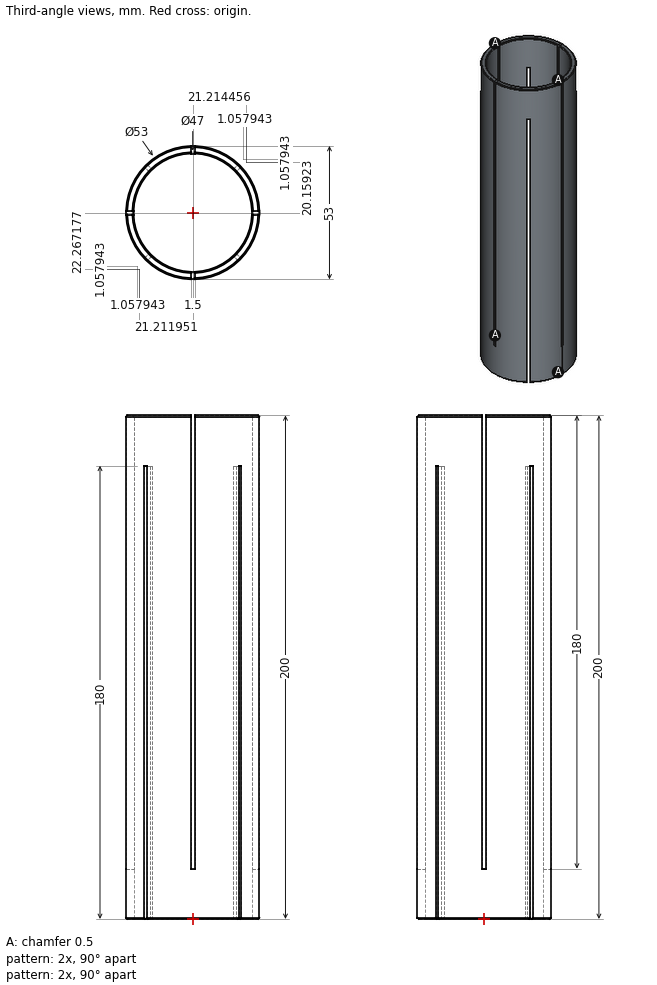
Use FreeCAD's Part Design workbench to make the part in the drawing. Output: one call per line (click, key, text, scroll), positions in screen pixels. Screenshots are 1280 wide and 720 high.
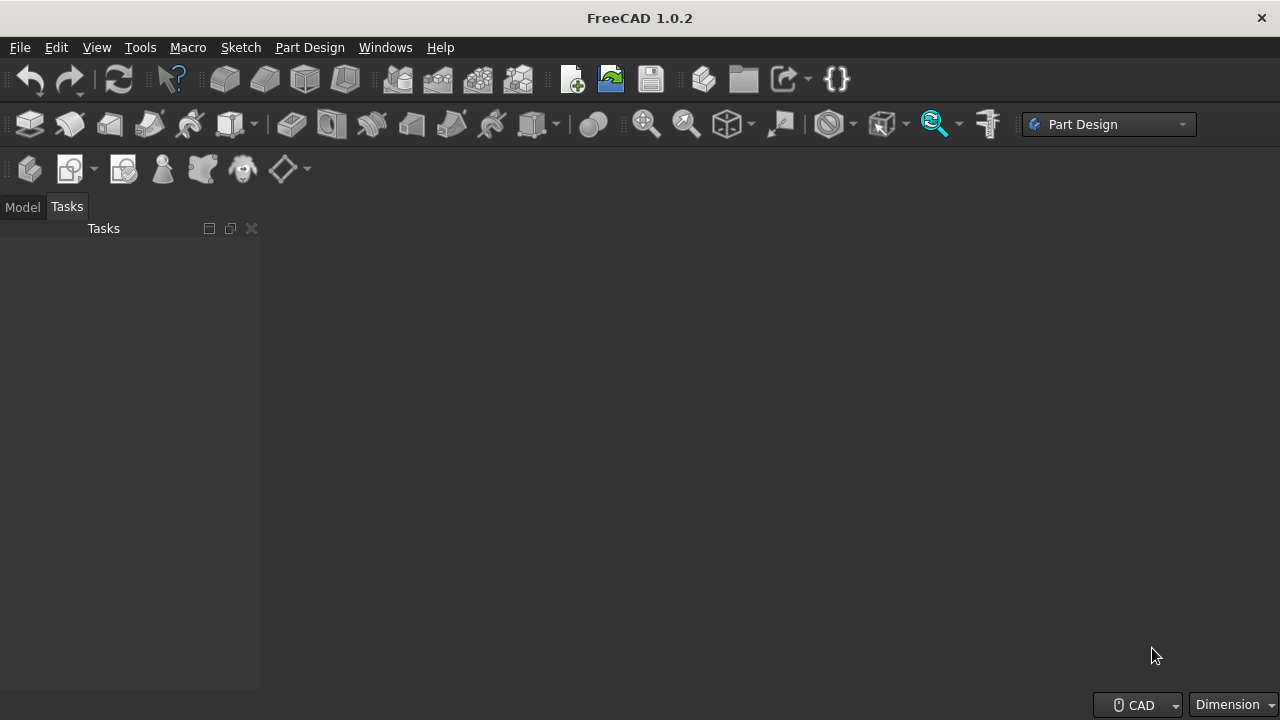
click(572, 80)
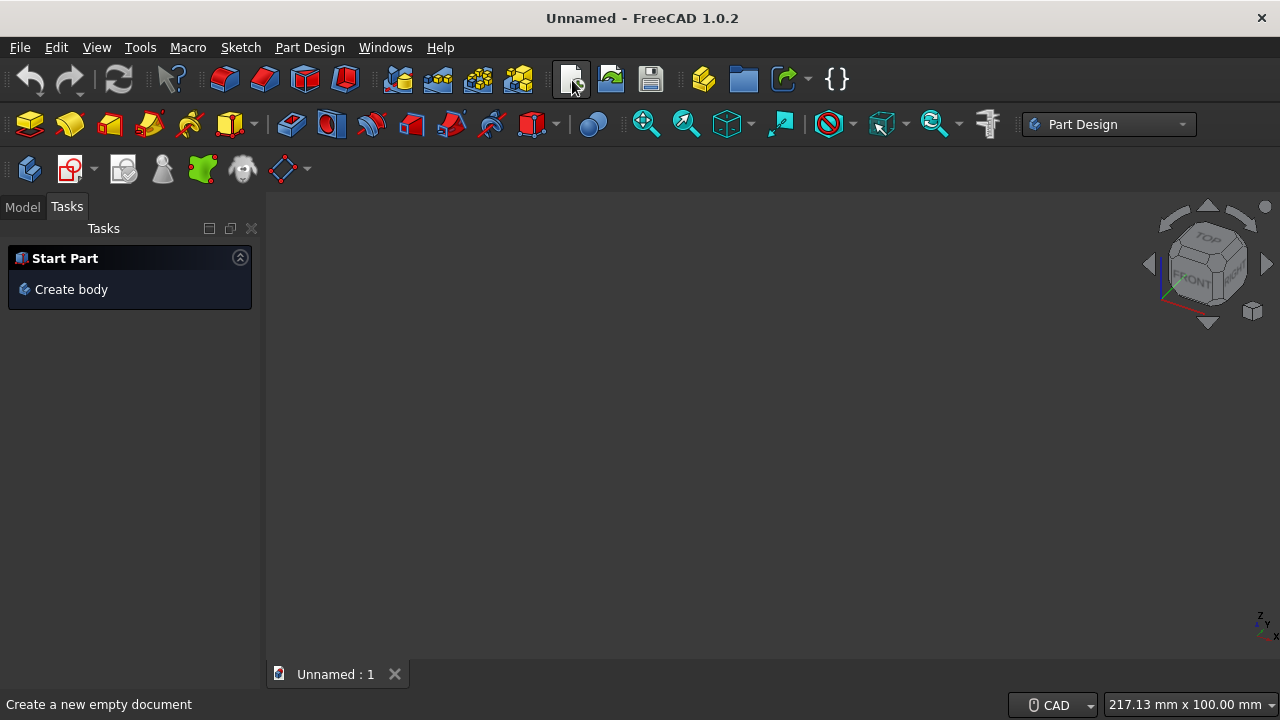
click(70, 170)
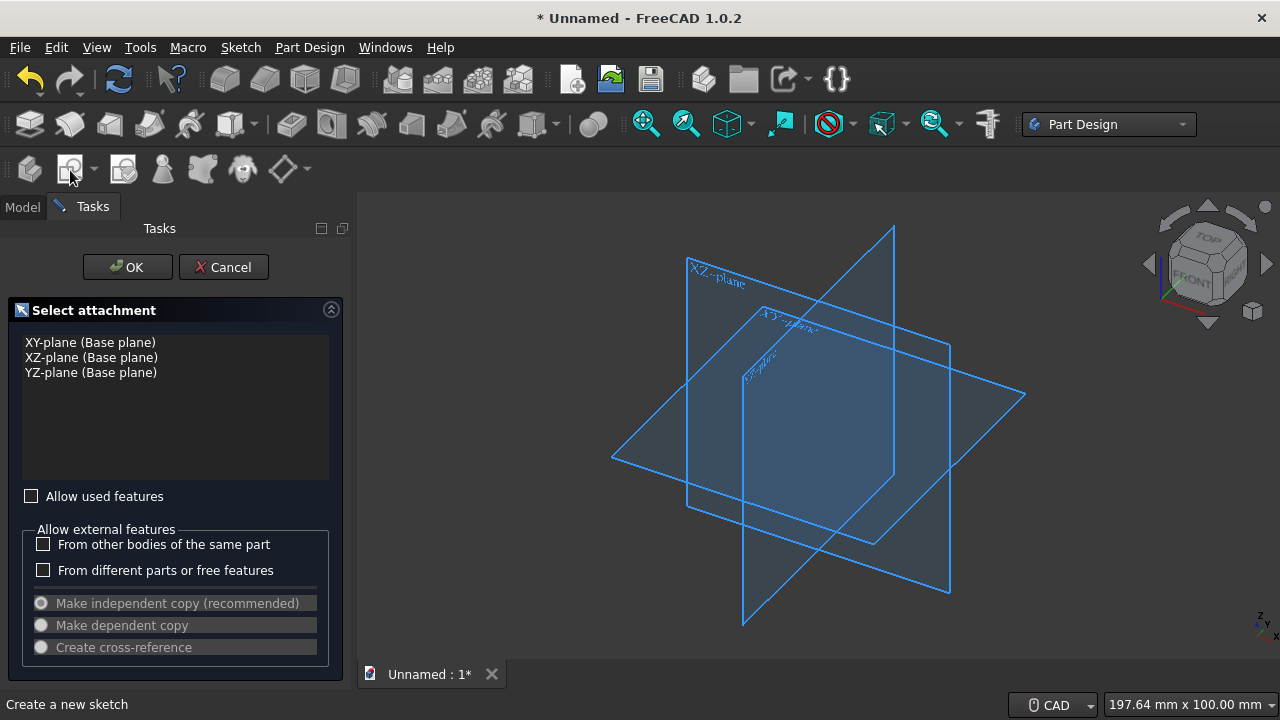
click(82, 342)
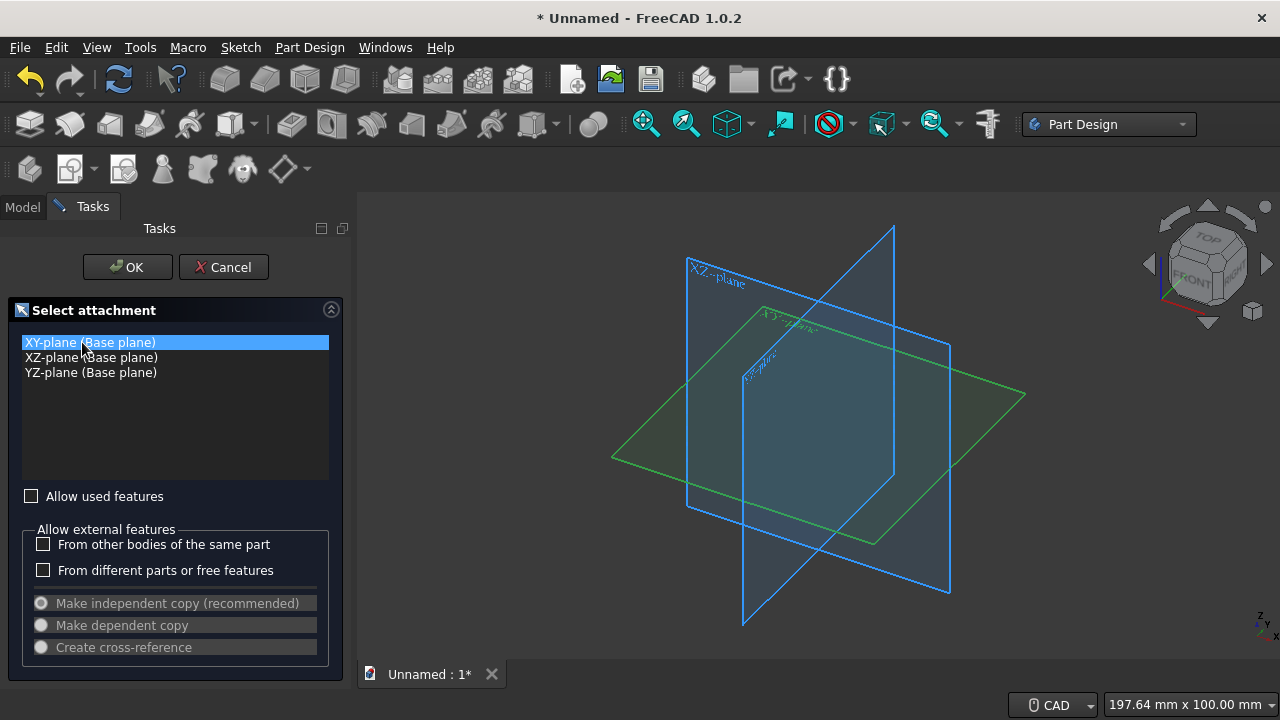
click(128, 267)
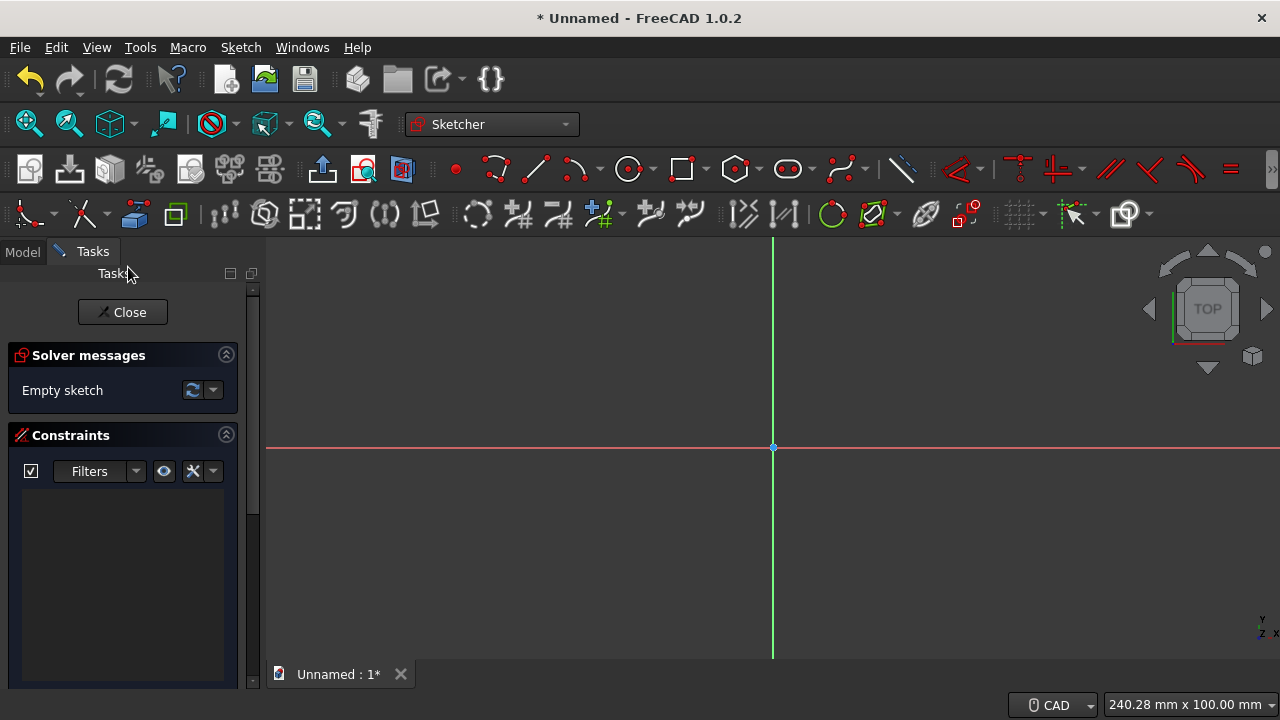
click(630, 170)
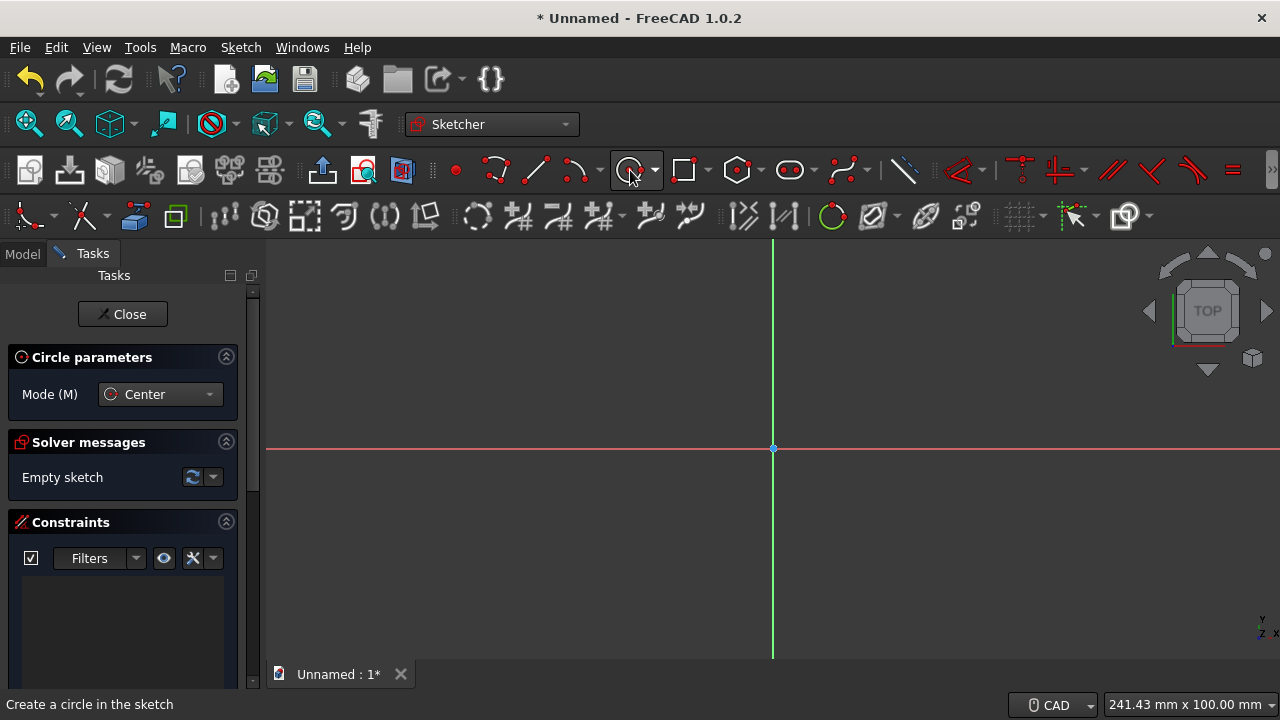
click(773, 449)
move(852, 370)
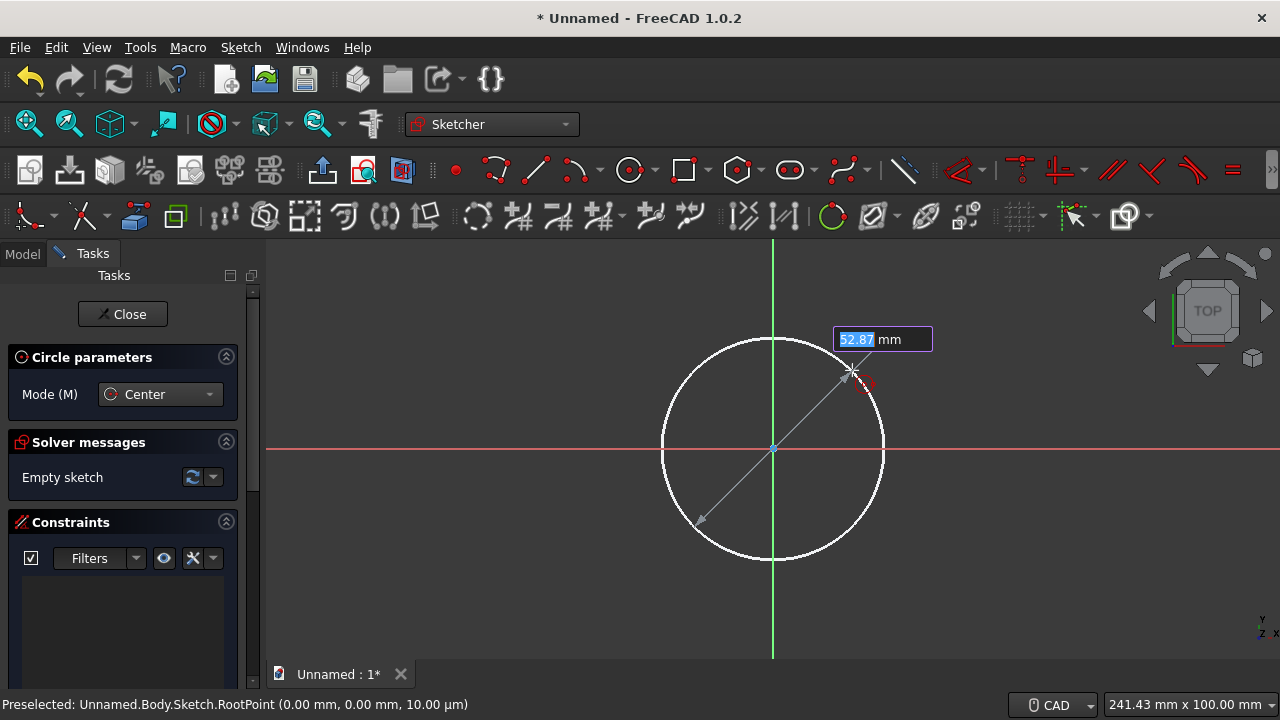
text(53)
key(Return)
key(Escape)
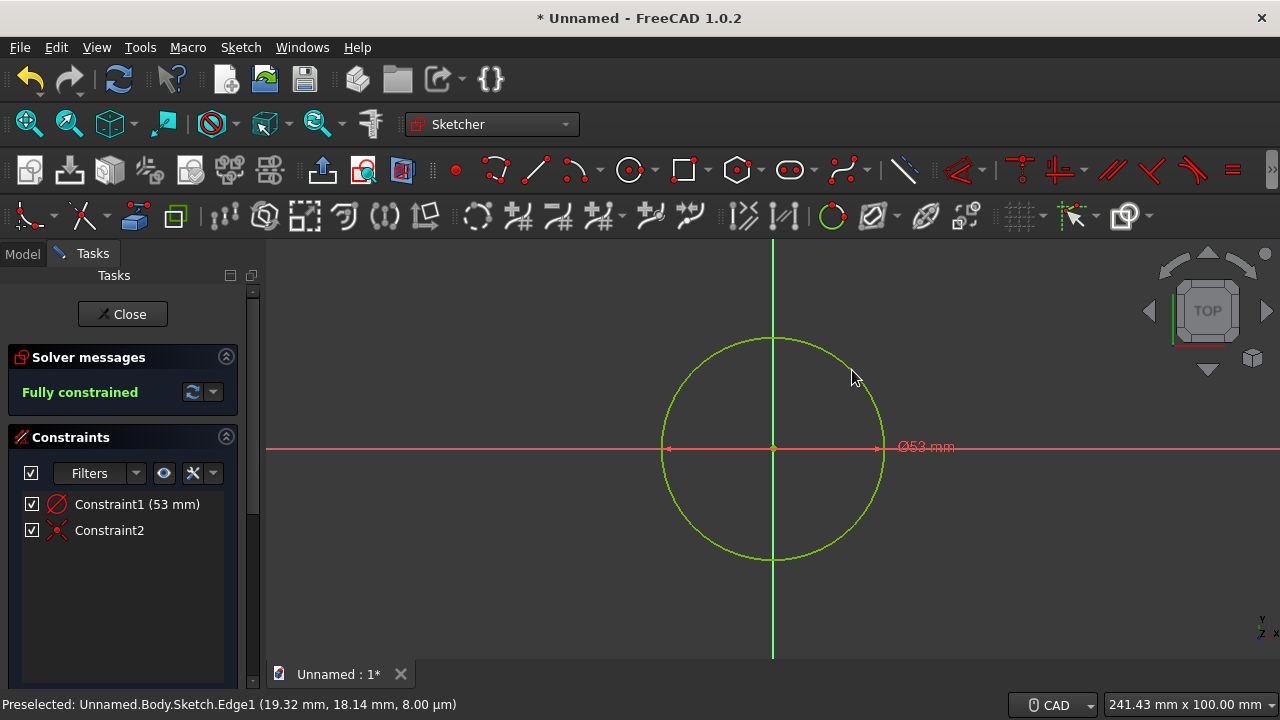
click(123, 314)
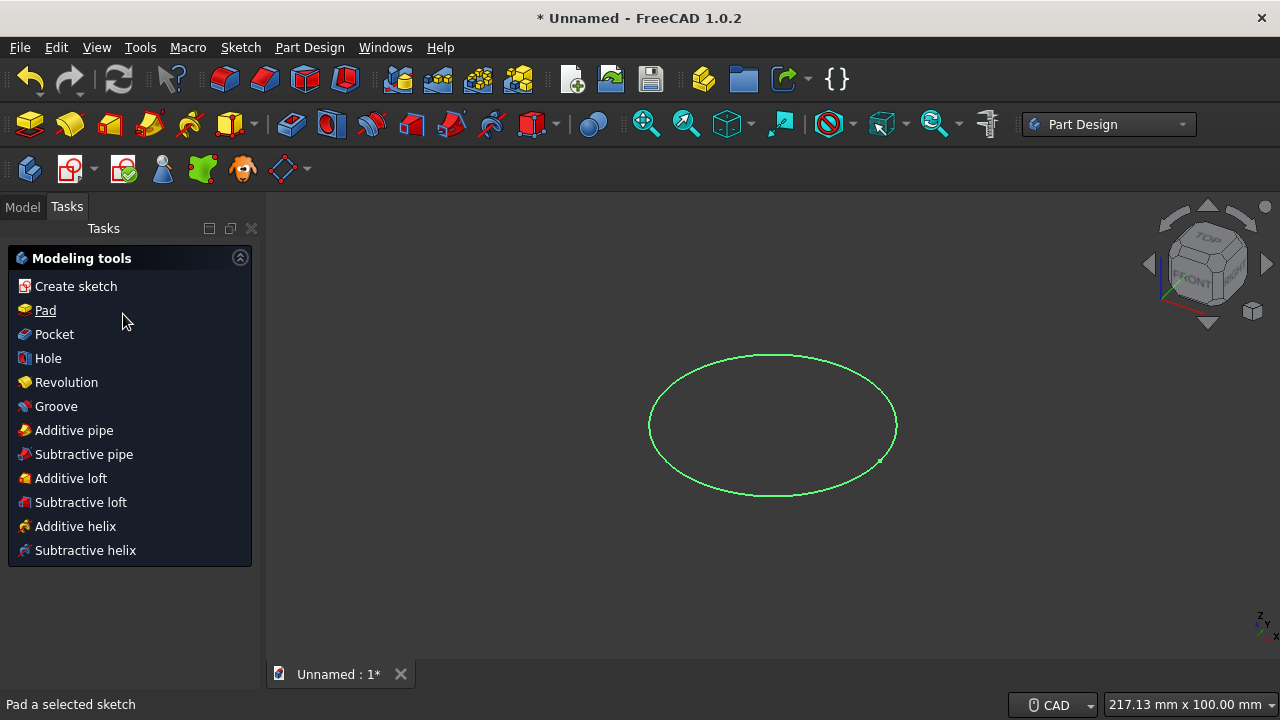
click(30, 124)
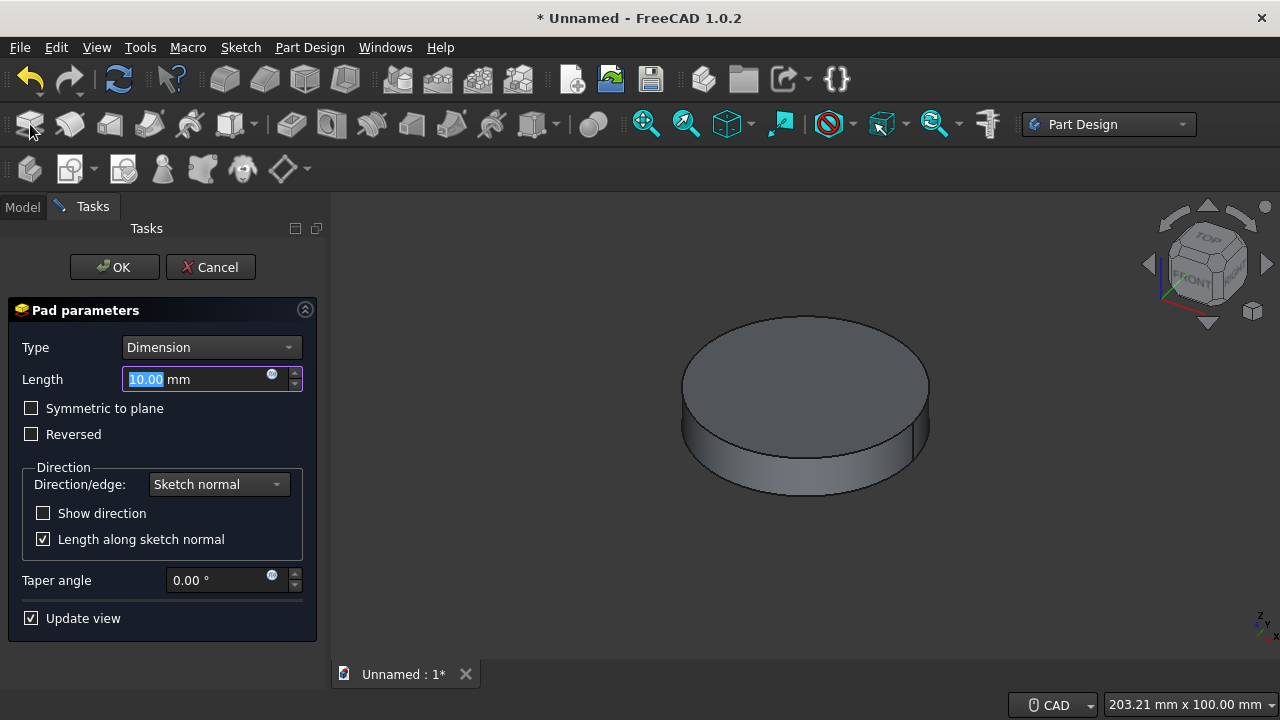
text(200)
key(Tab)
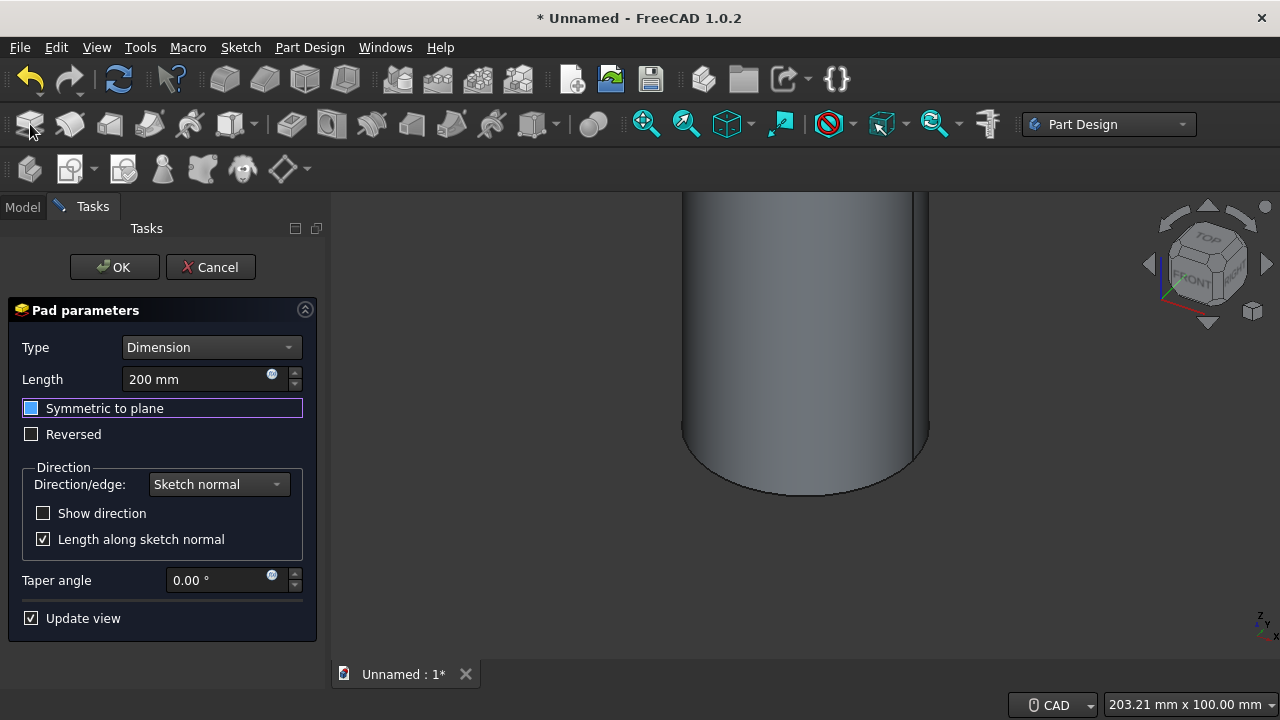
click(115, 267)